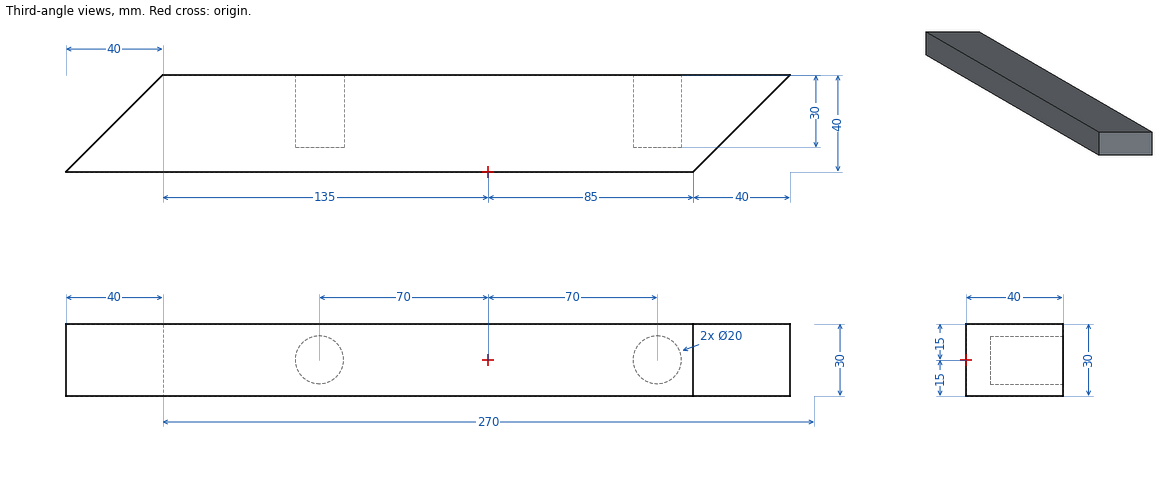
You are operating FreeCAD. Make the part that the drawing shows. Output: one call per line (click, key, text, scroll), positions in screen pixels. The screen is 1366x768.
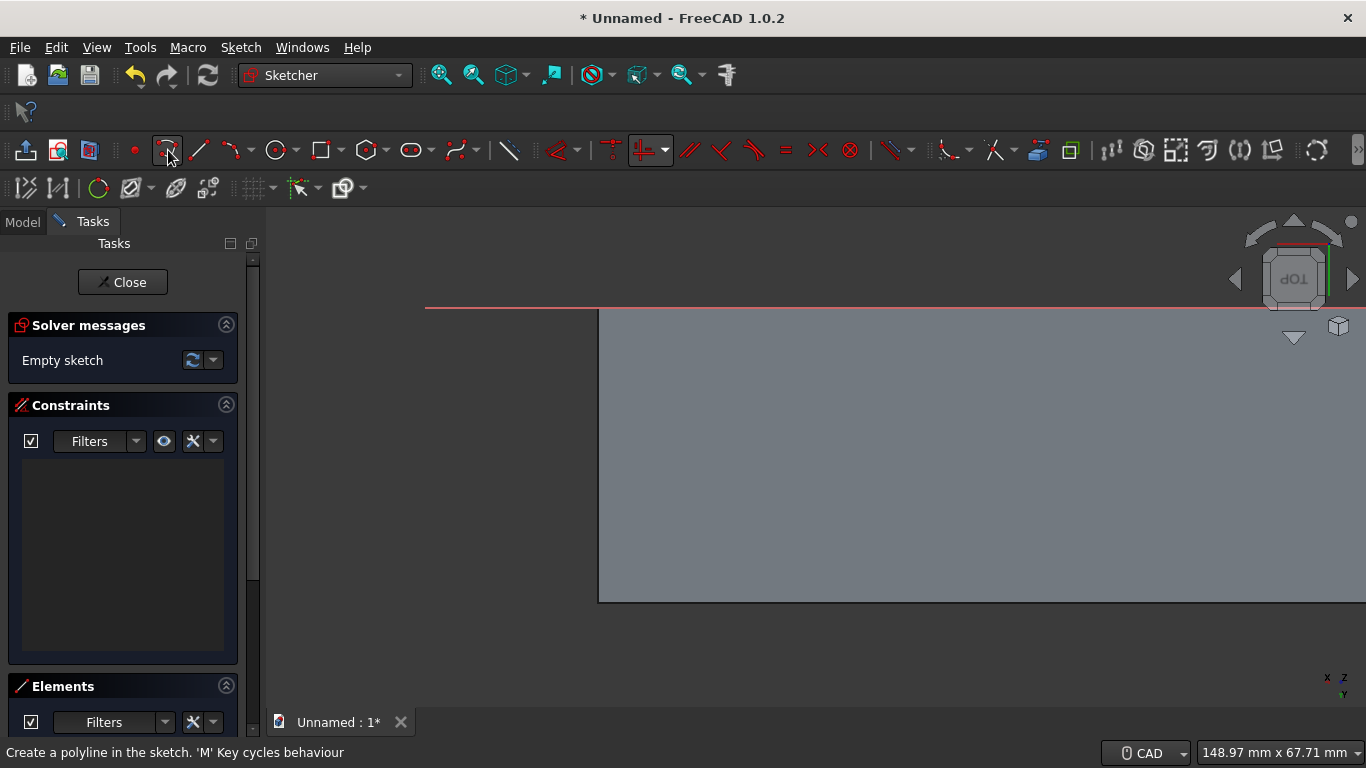
click(893, 308)
click(598, 317)
click(598, 603)
click(893, 308)
key(Escape)
key(Escape)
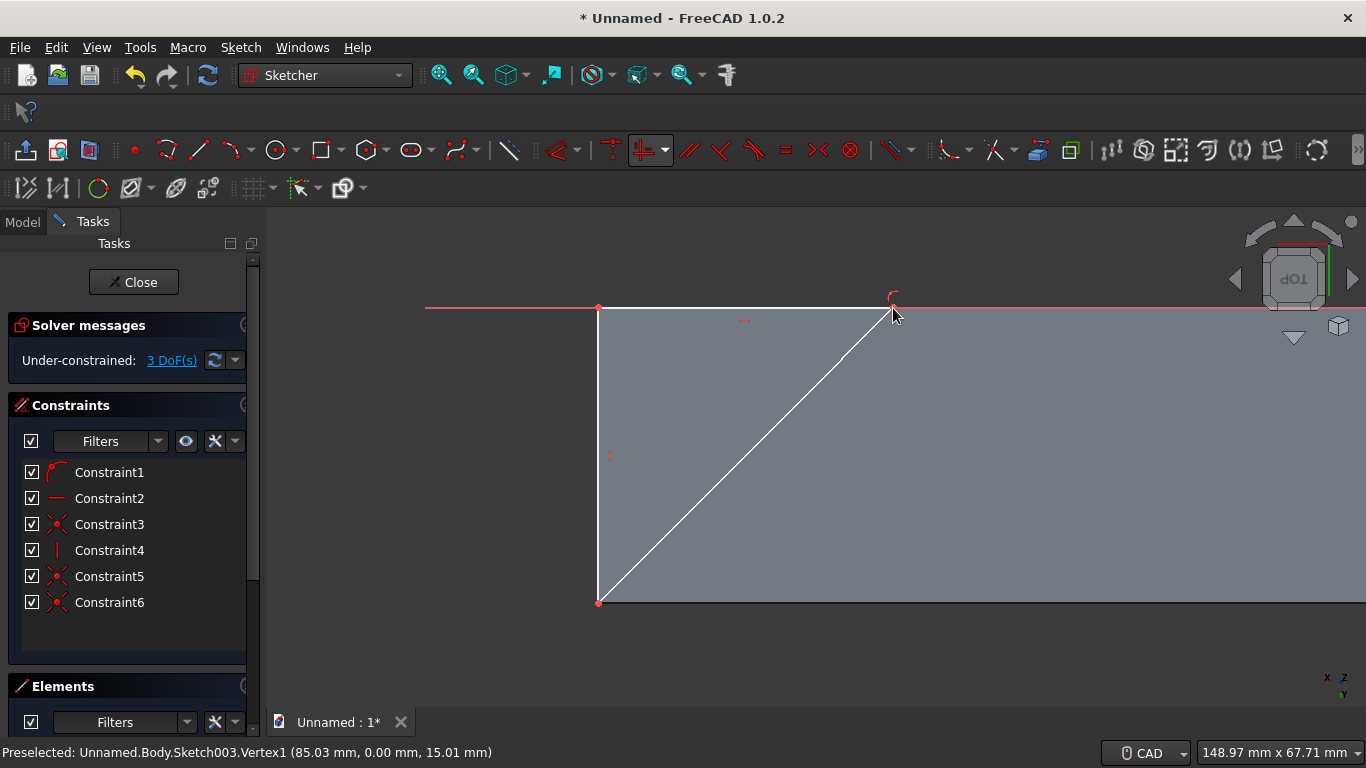
click(556, 150)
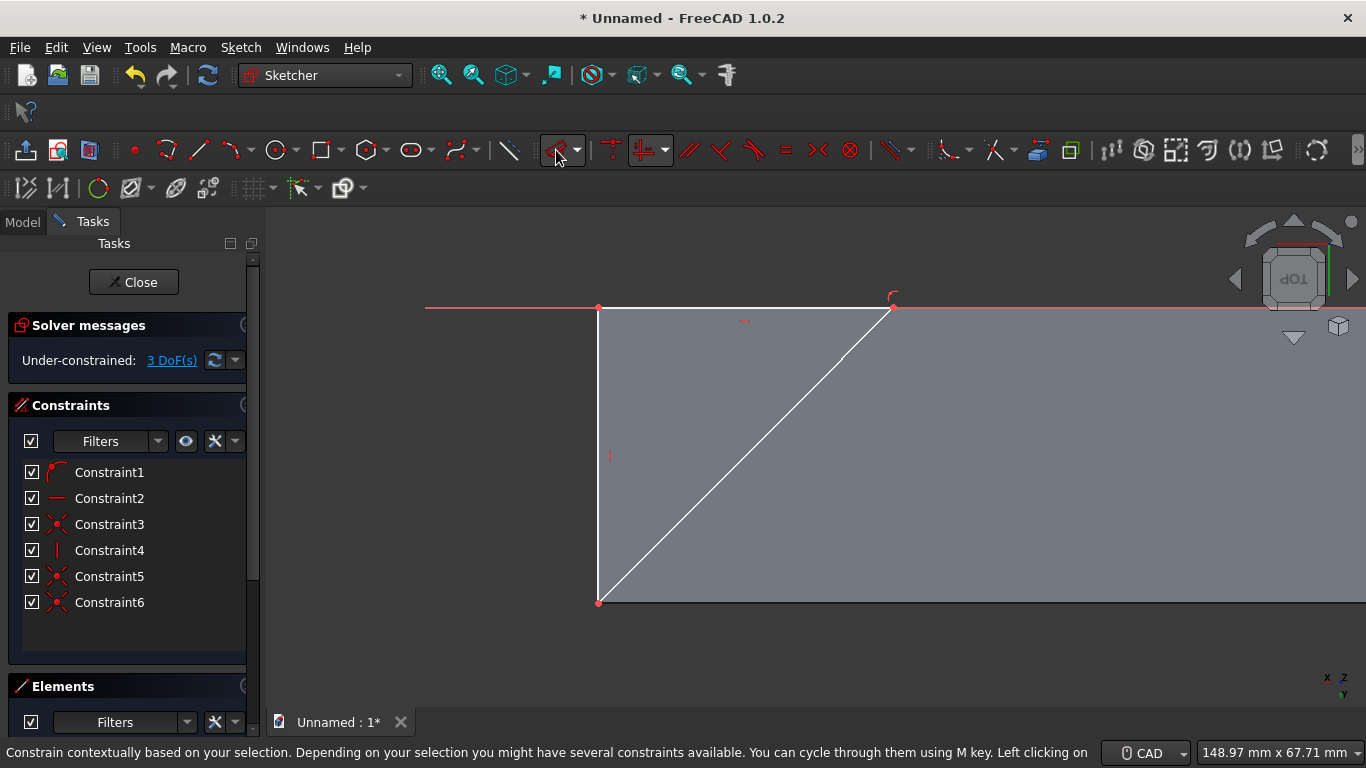
click(804, 308)
click(745, 274)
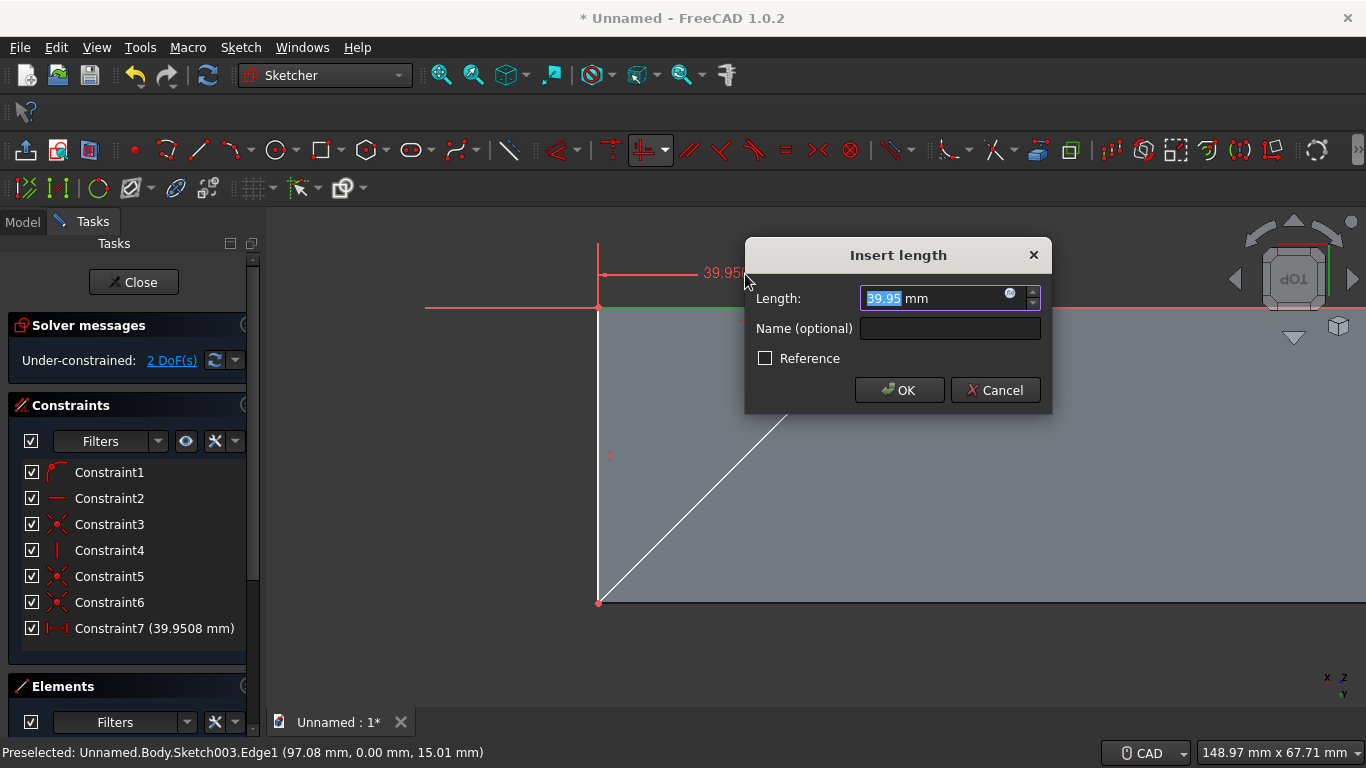
text(40)
key(Return)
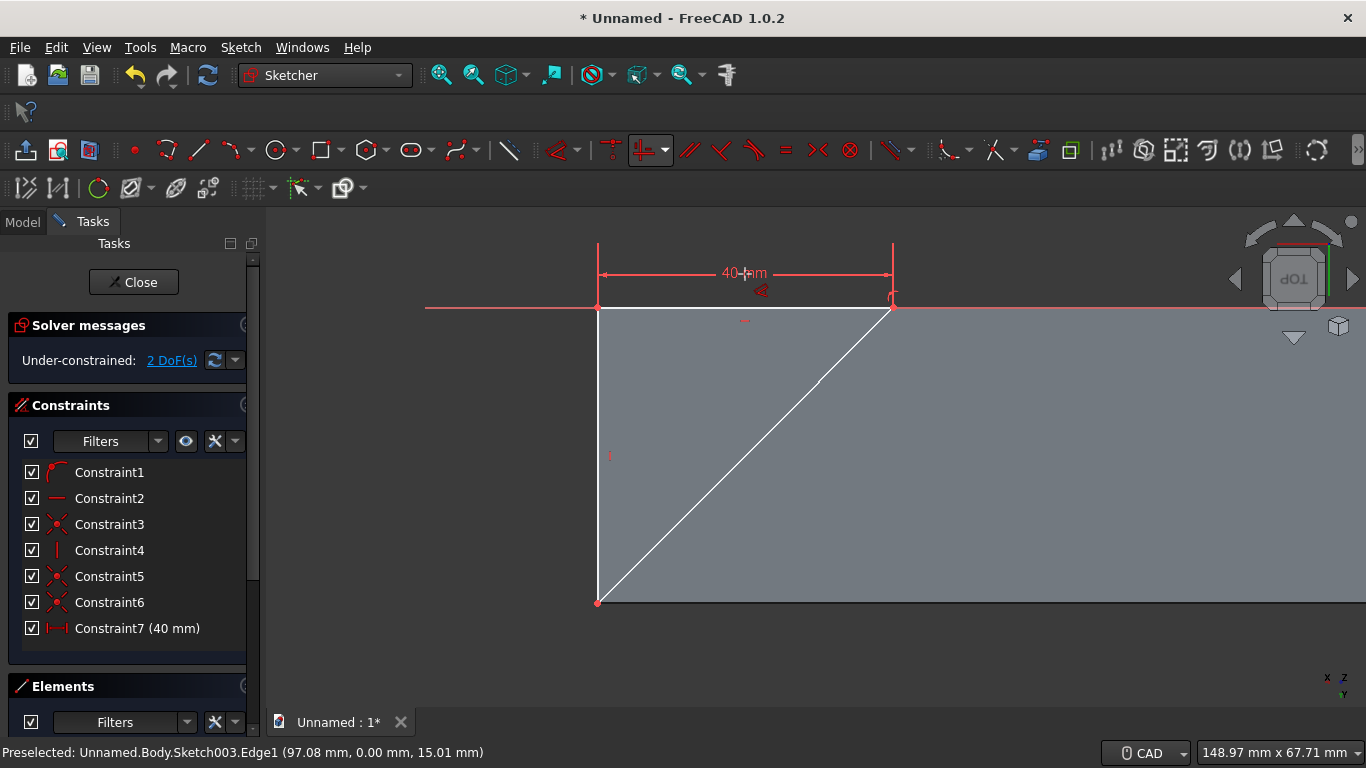
click(598, 397)
click(564, 456)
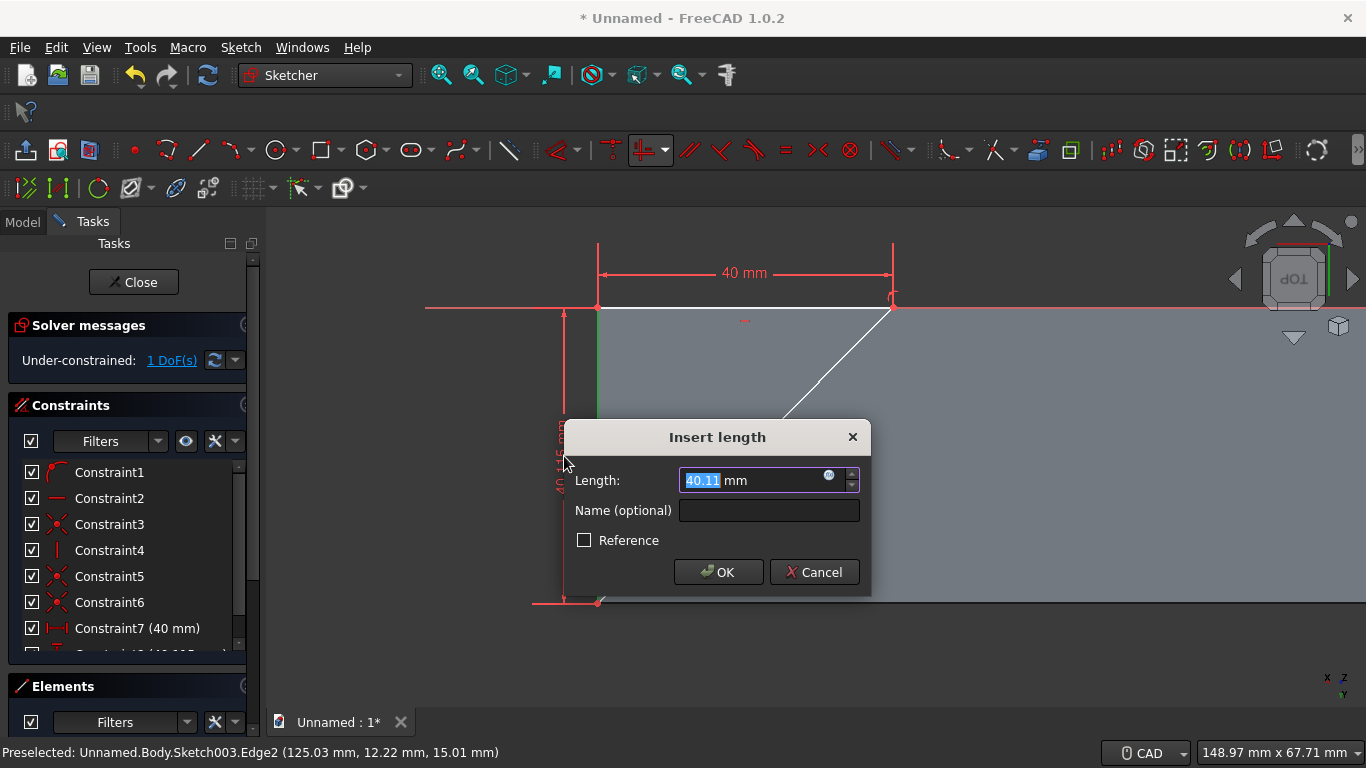
text(40)
key(Return)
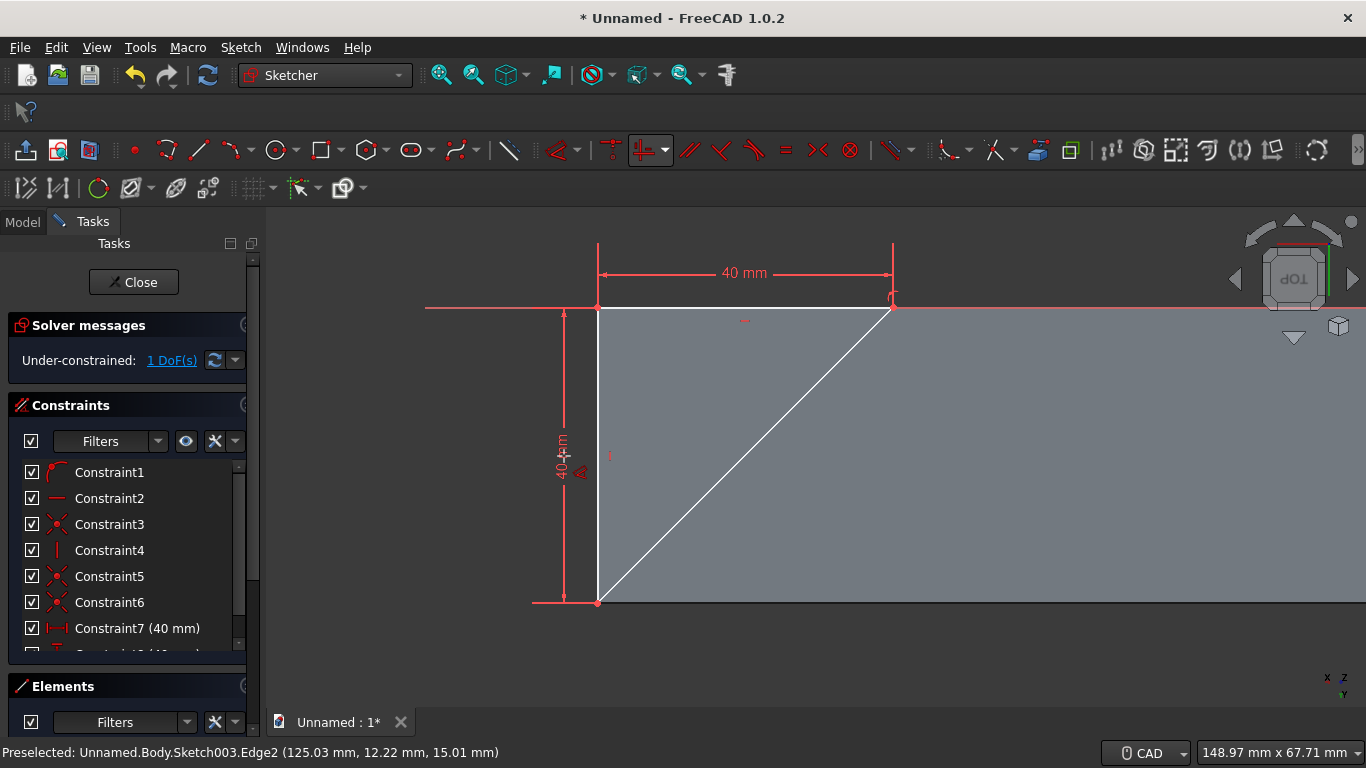
click(893, 308)
click(1047, 274)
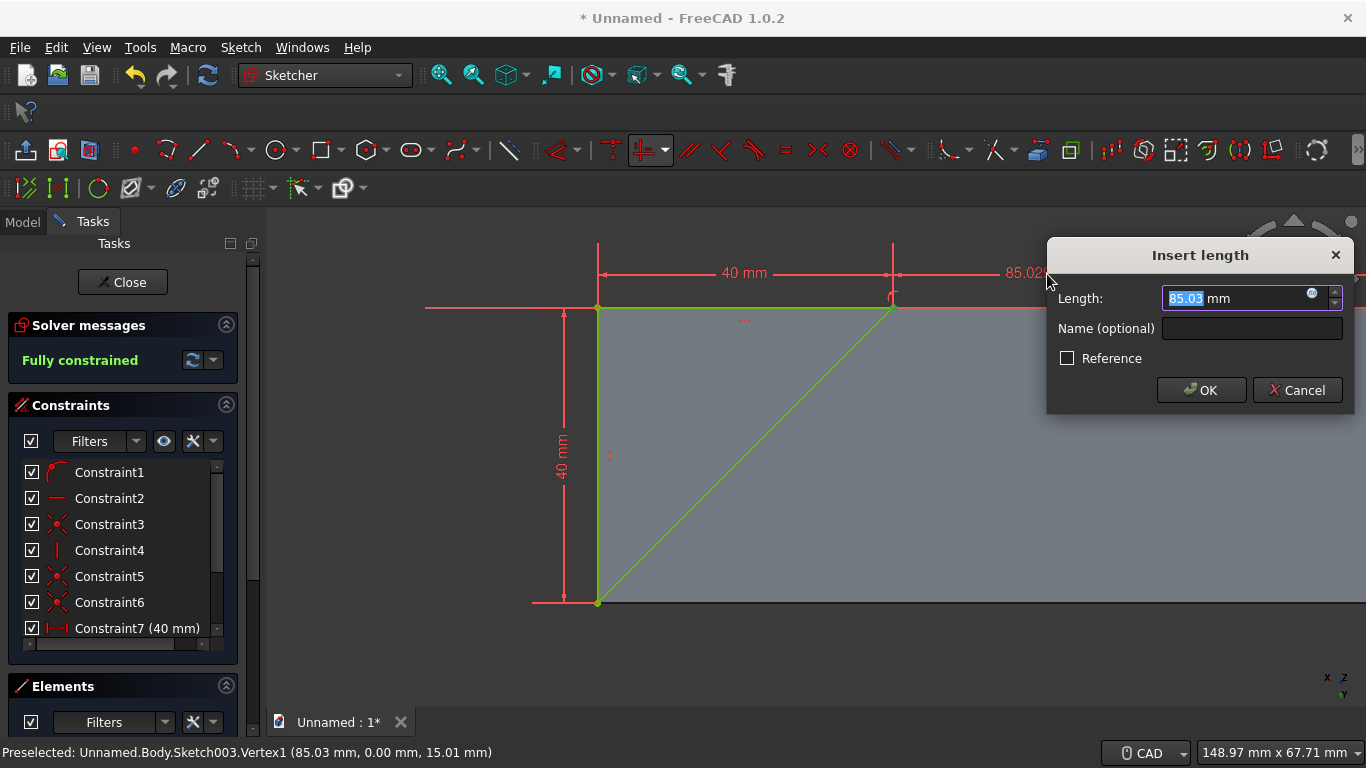
text(85)
key(Return)
key(Escape)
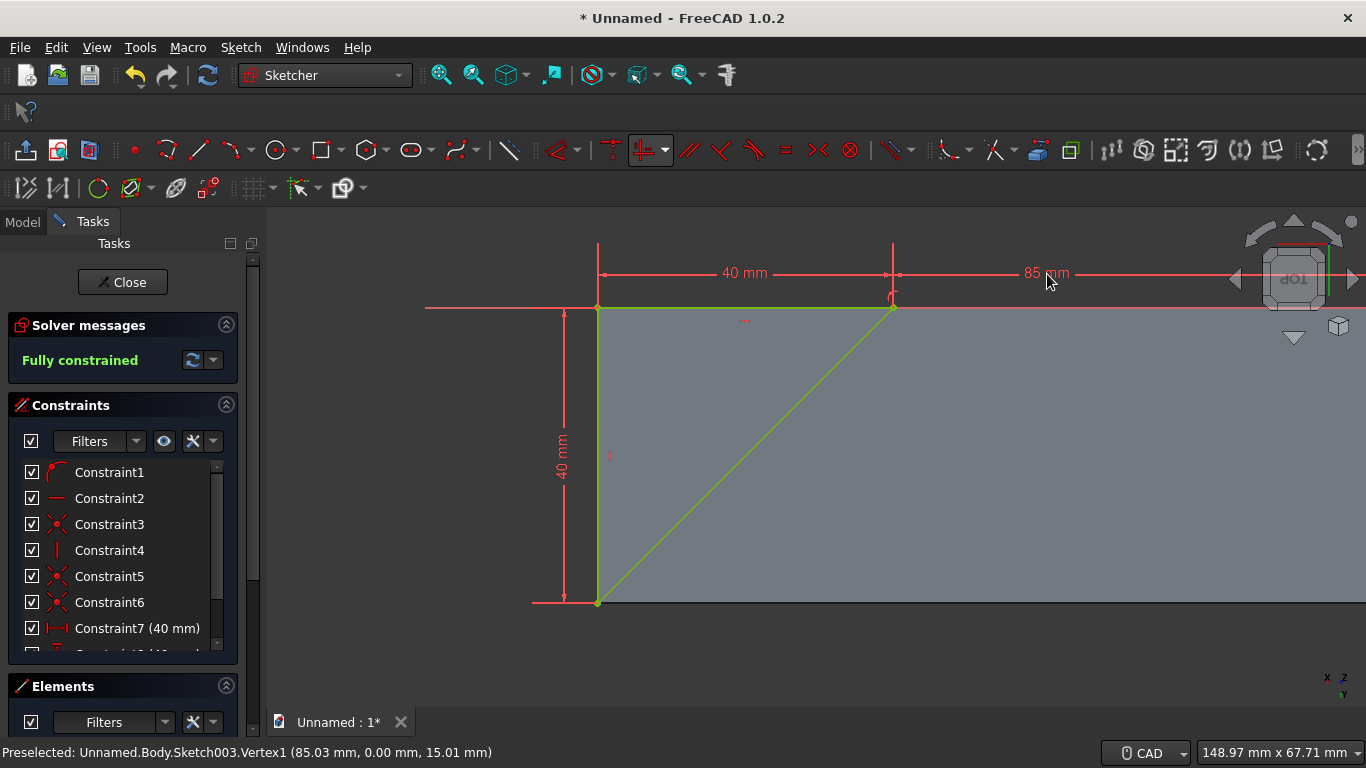
click(123, 282)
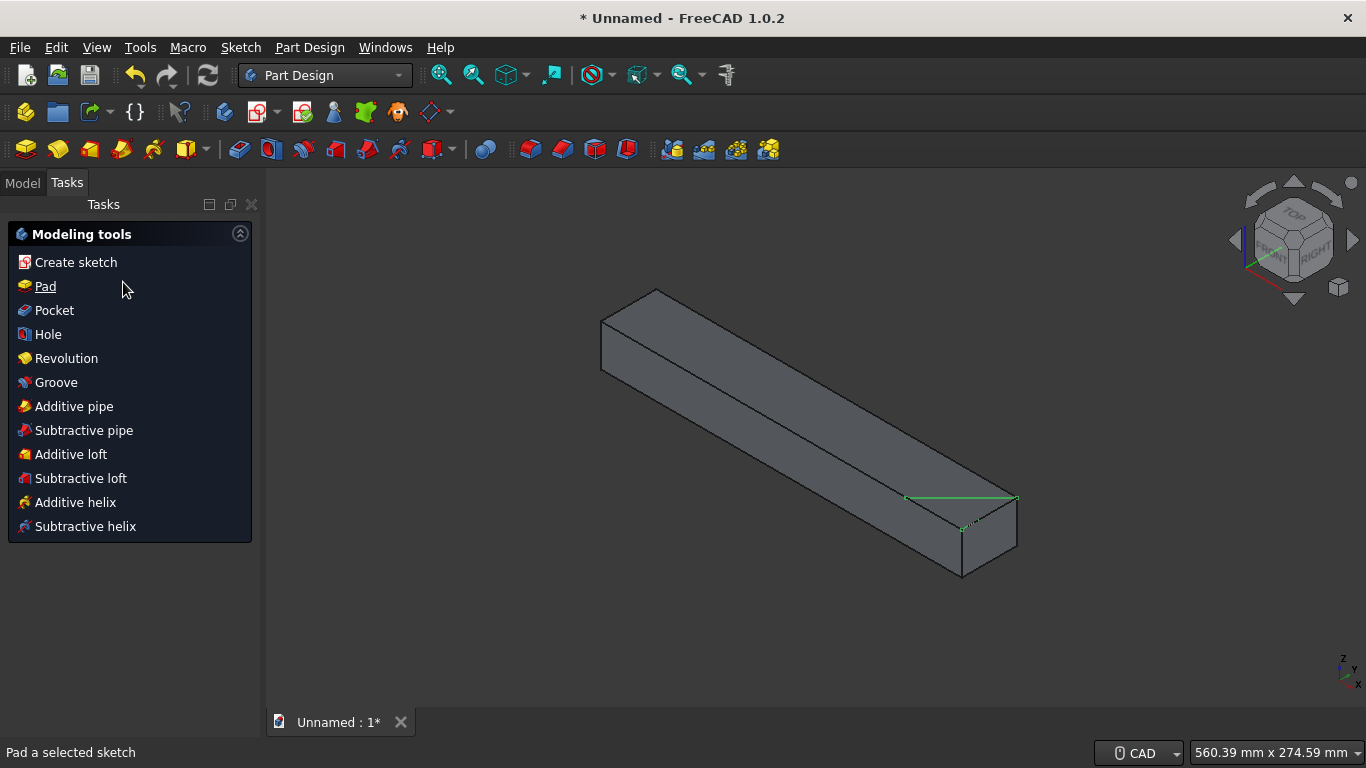
click(240, 150)